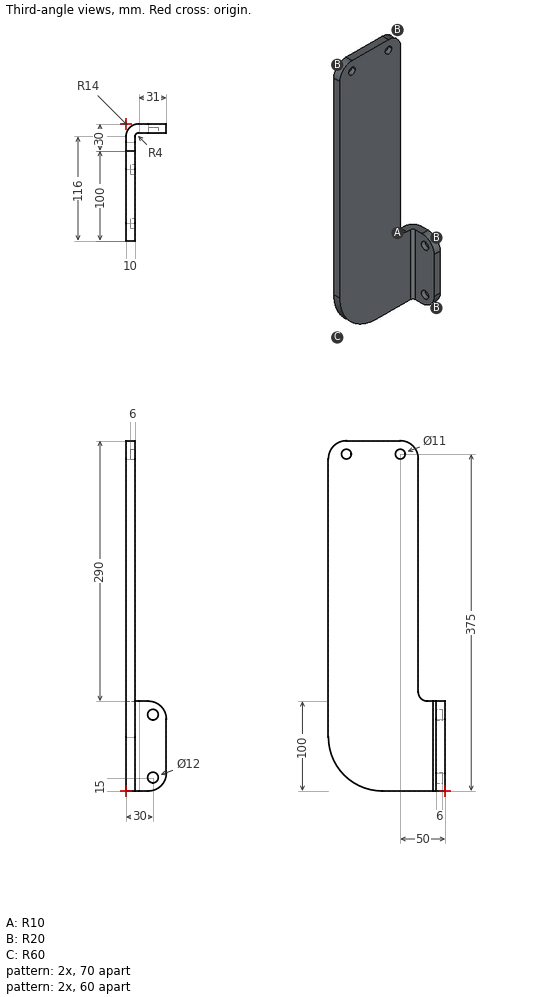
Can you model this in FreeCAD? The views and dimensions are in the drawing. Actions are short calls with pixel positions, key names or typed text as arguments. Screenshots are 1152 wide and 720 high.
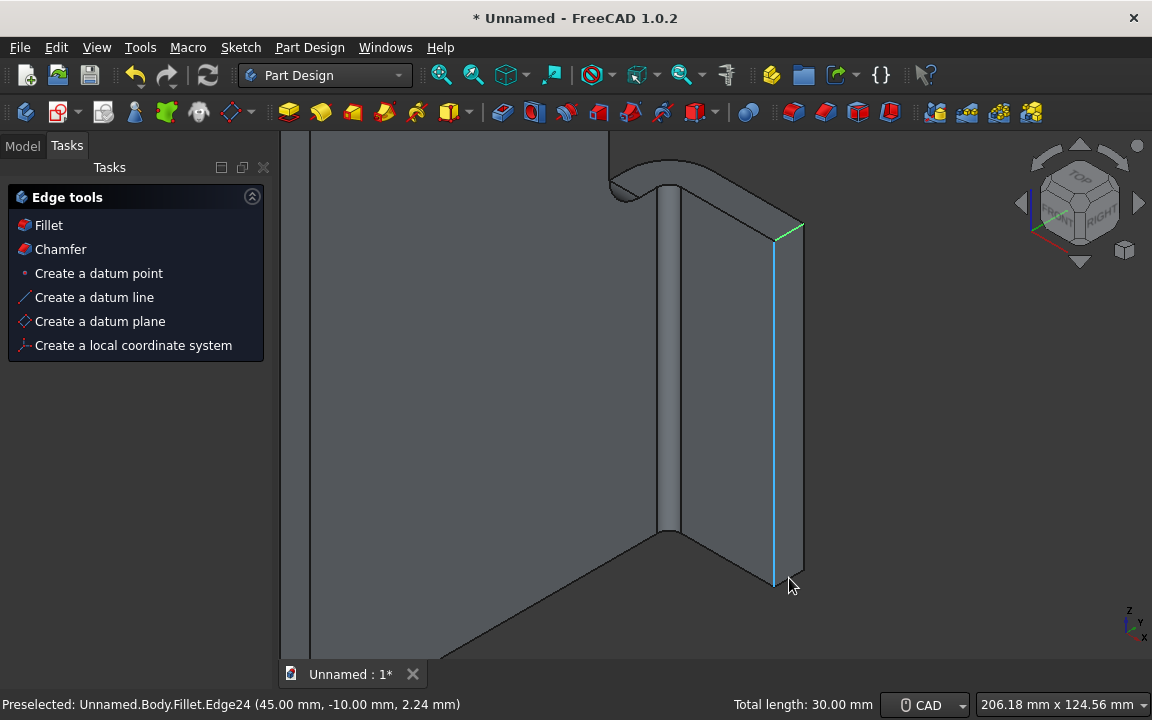
click(442, 76)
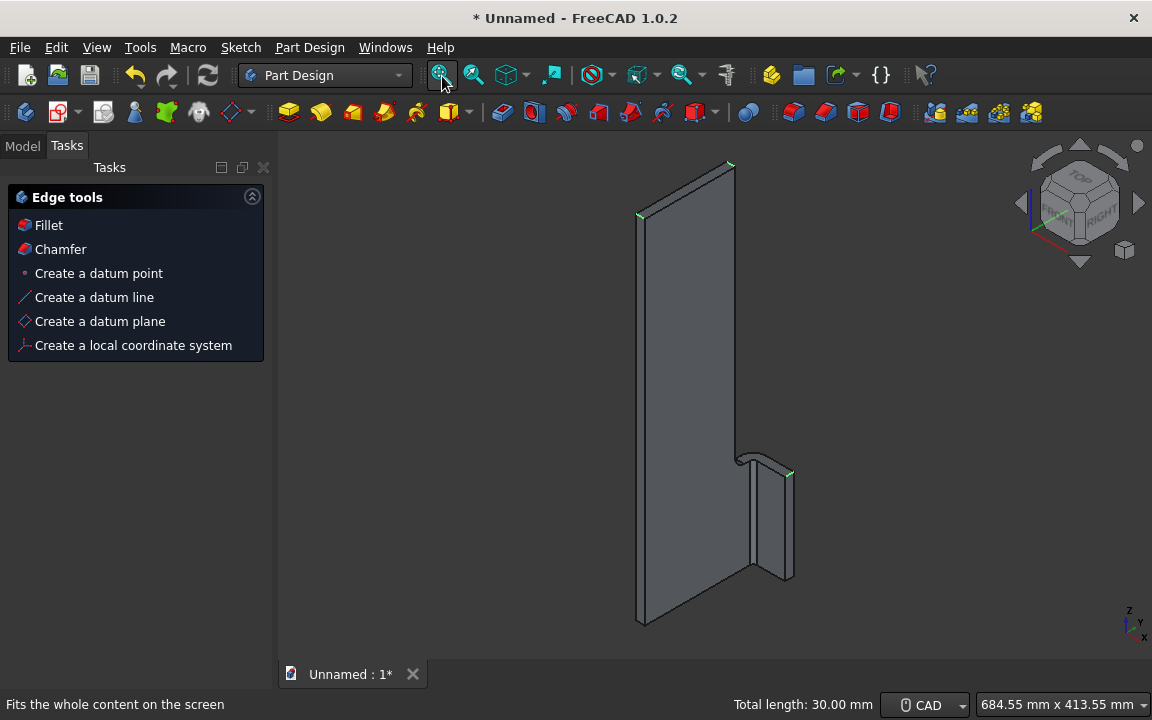
key(1)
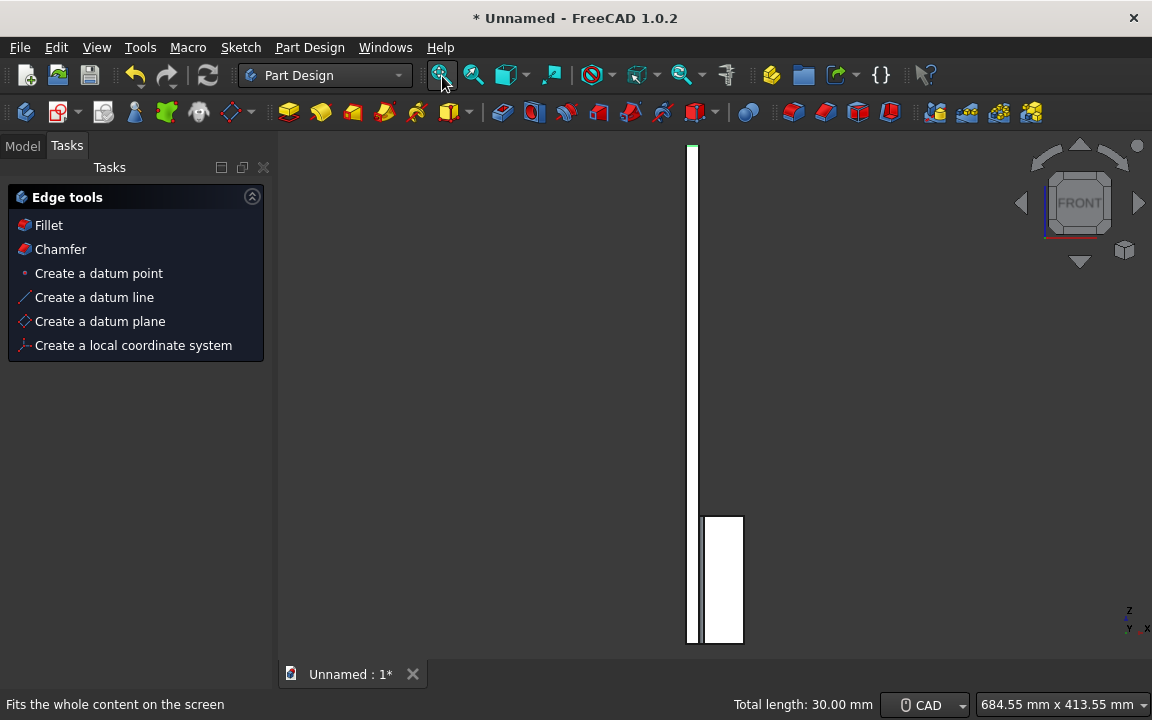
key(3)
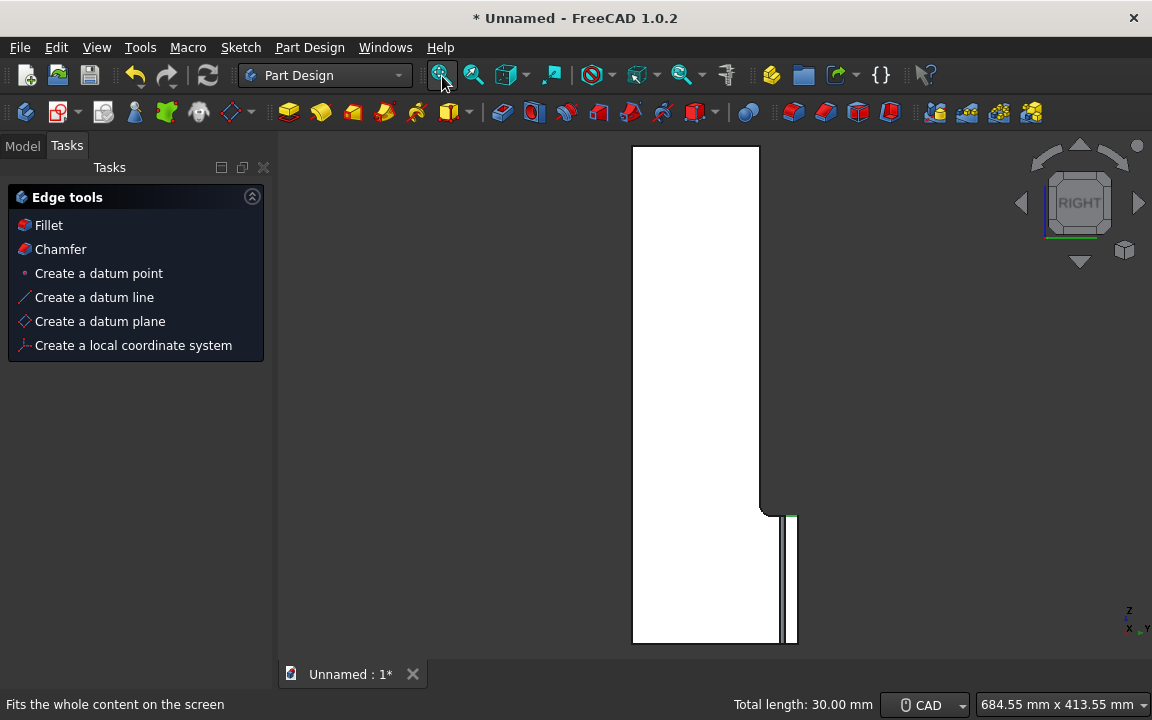
key(5)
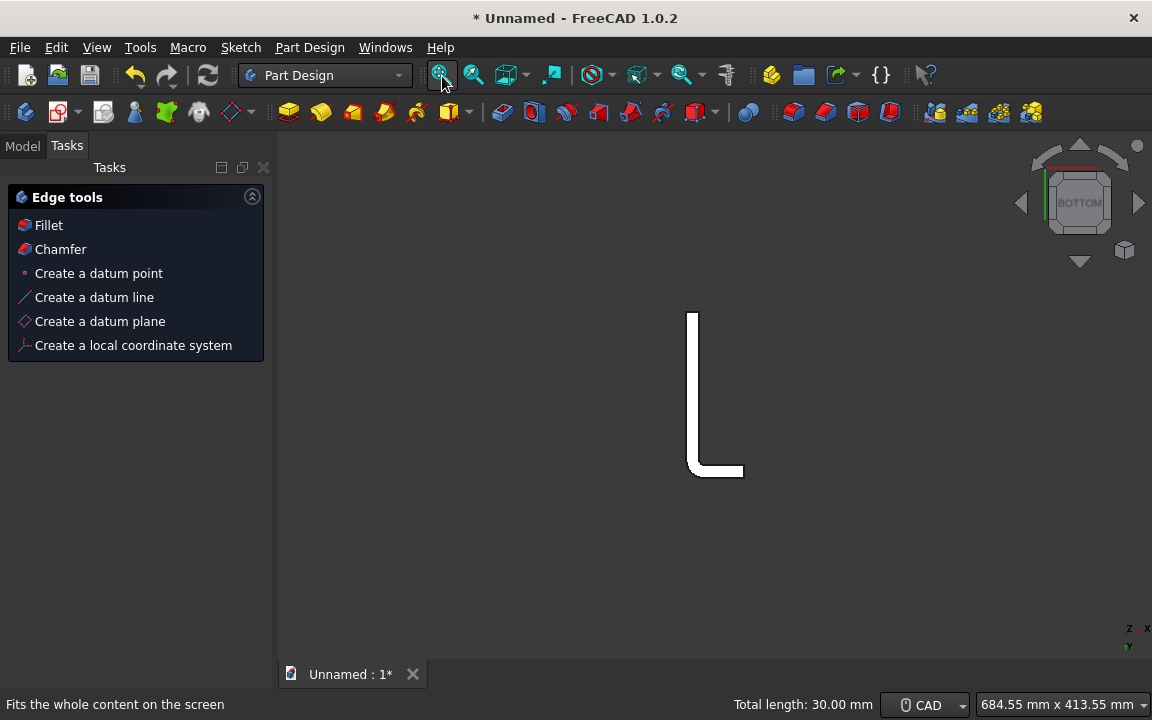
click(442, 76)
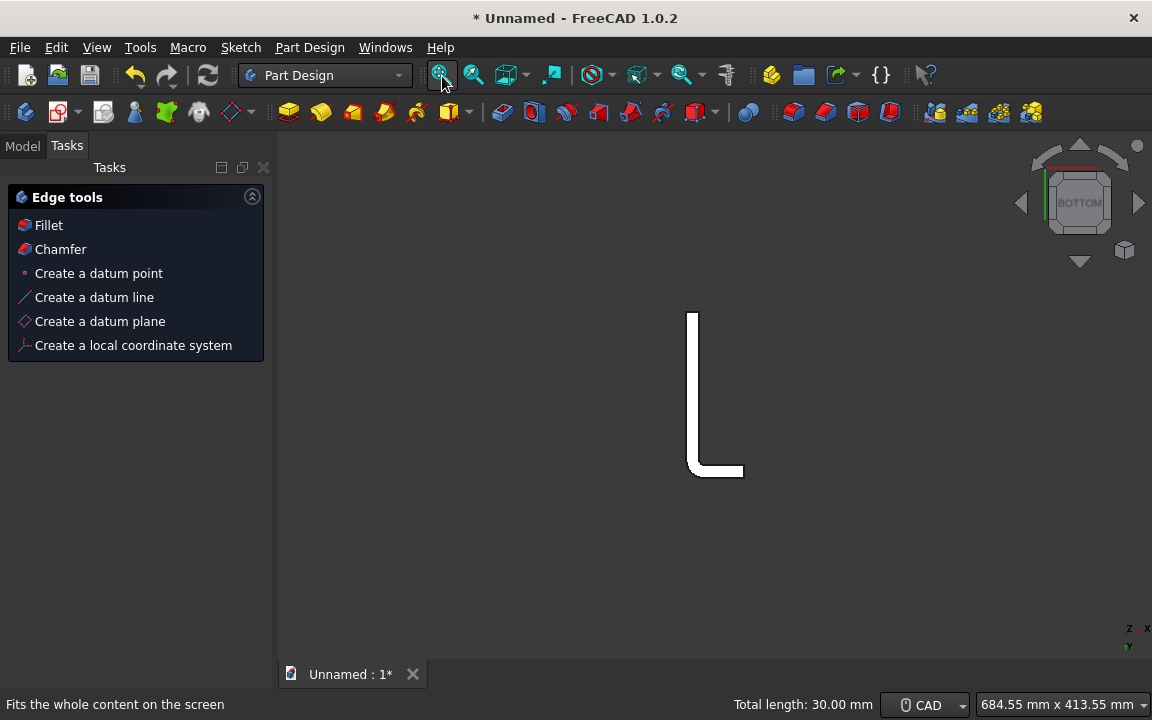
click(744, 471, ctrl)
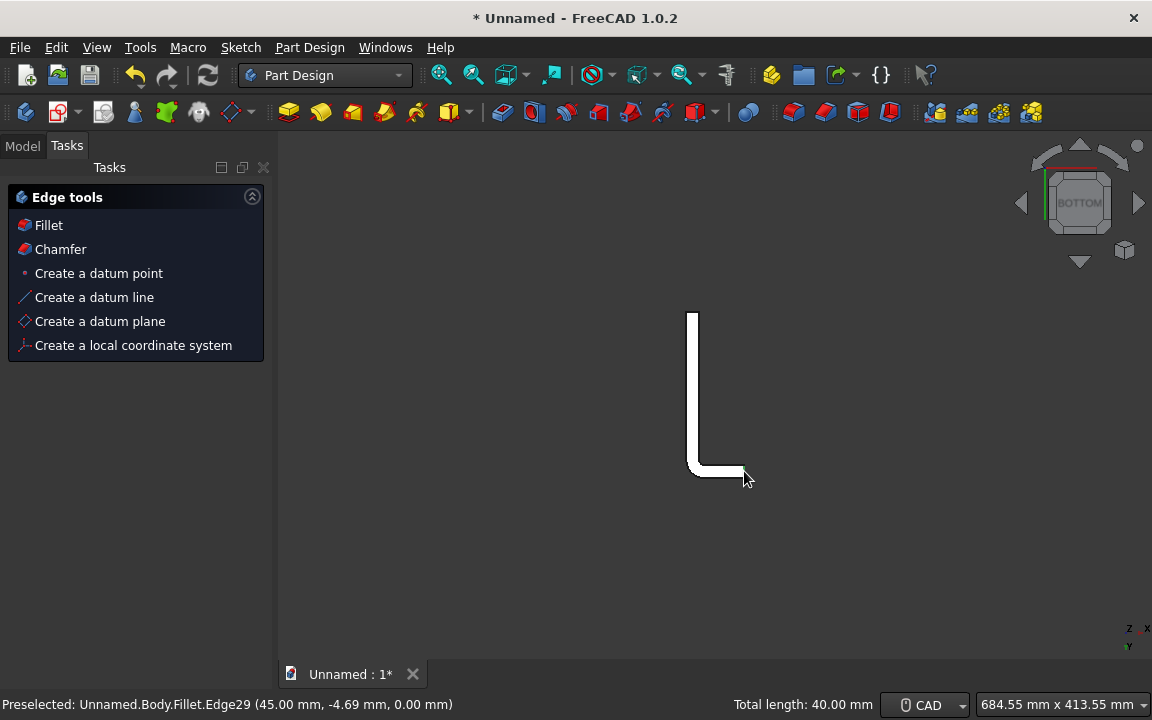
click(794, 112)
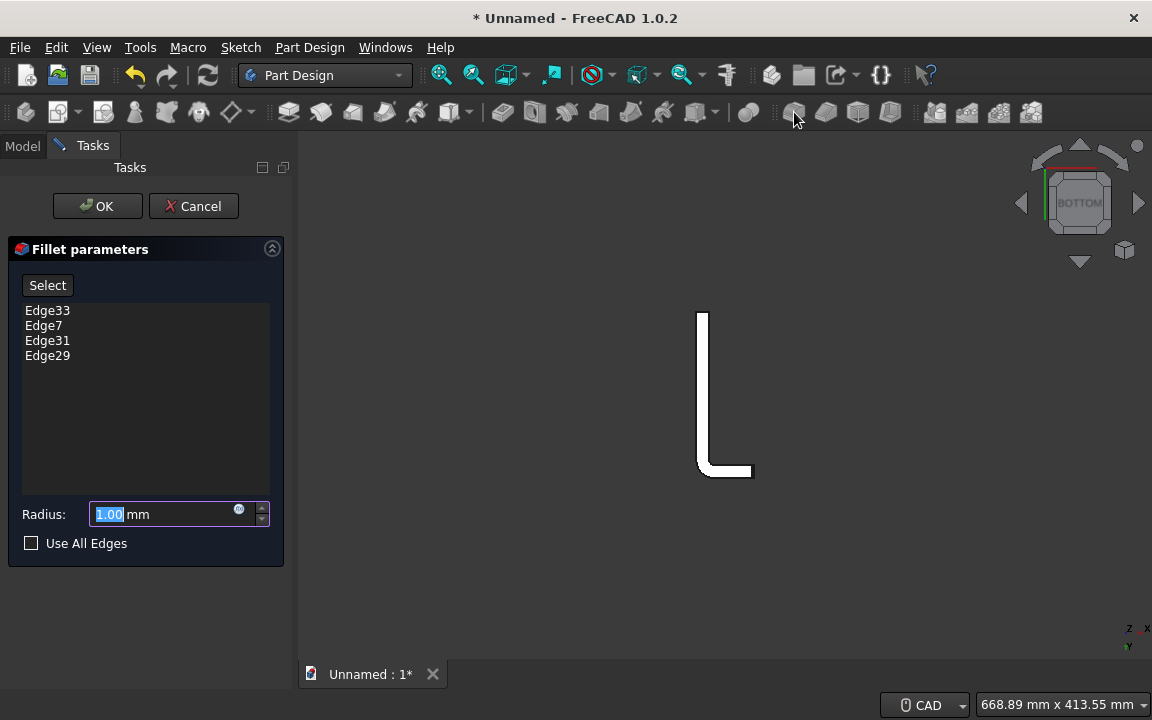
text(20)
key(Tab)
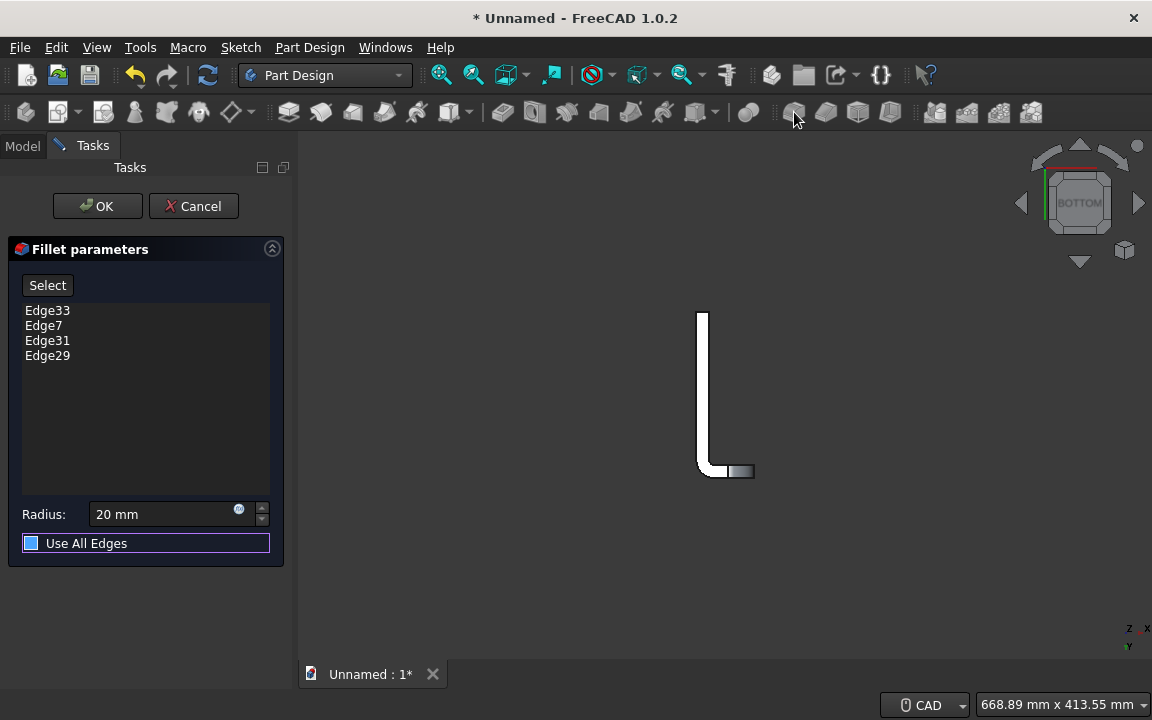
click(98, 206)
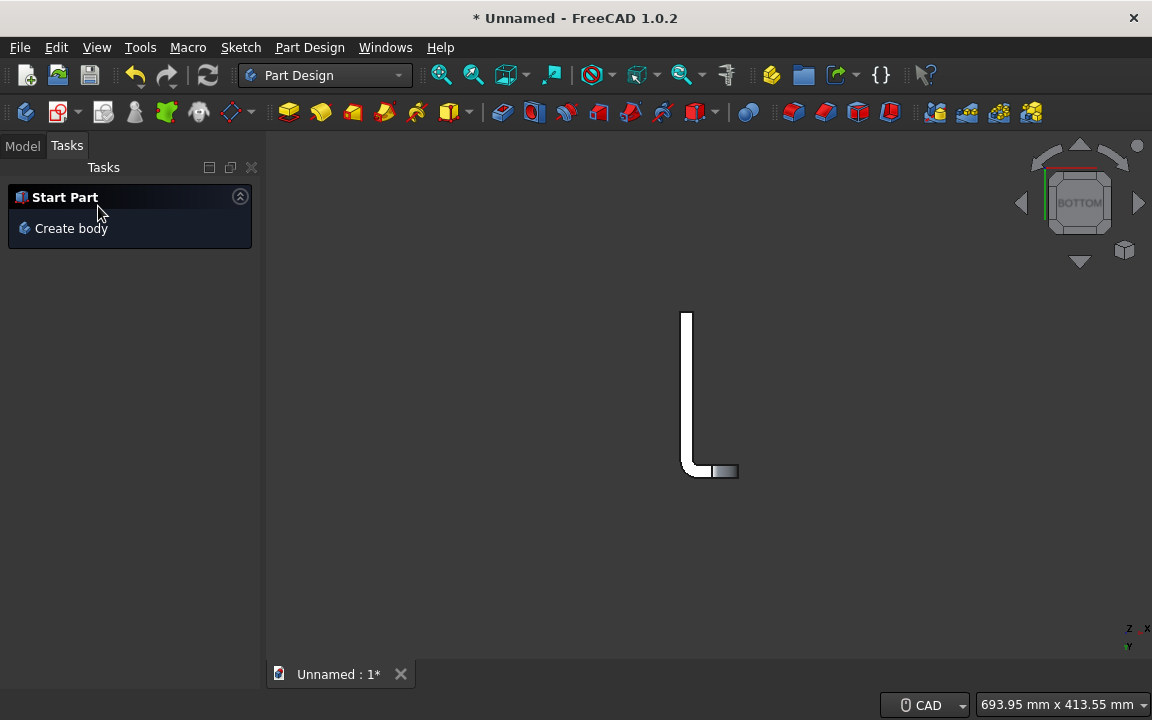
click(442, 76)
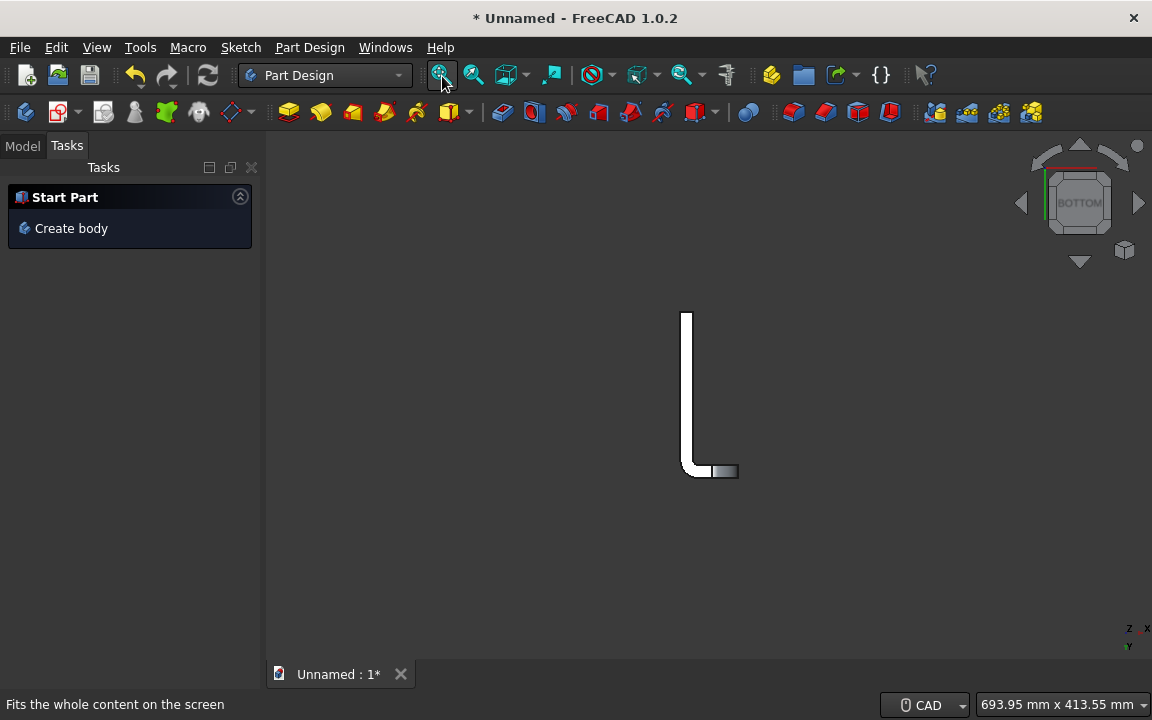
click(687, 311)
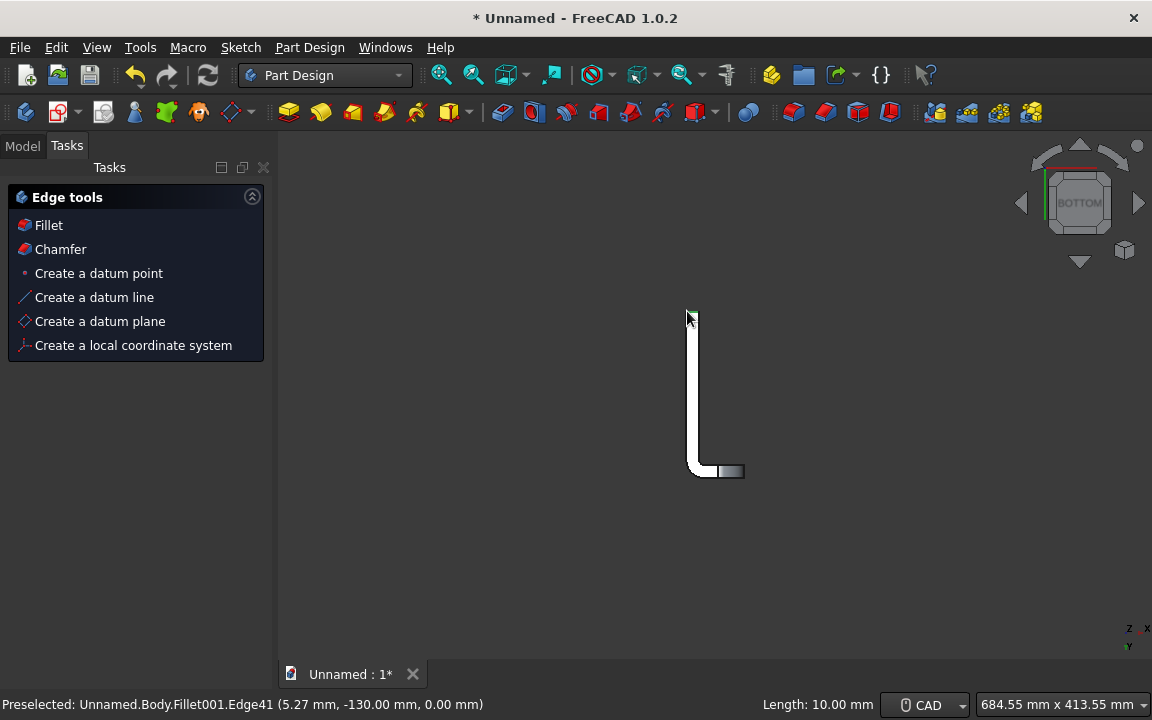
click(794, 112)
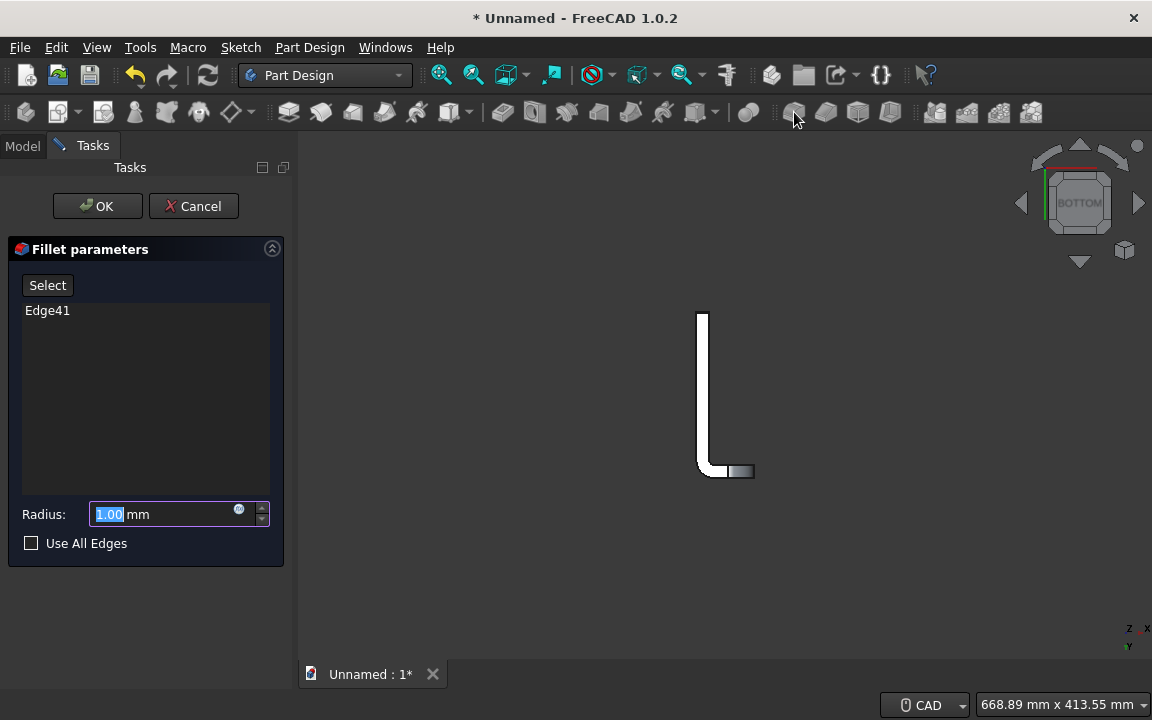
text(60)
key(Tab)